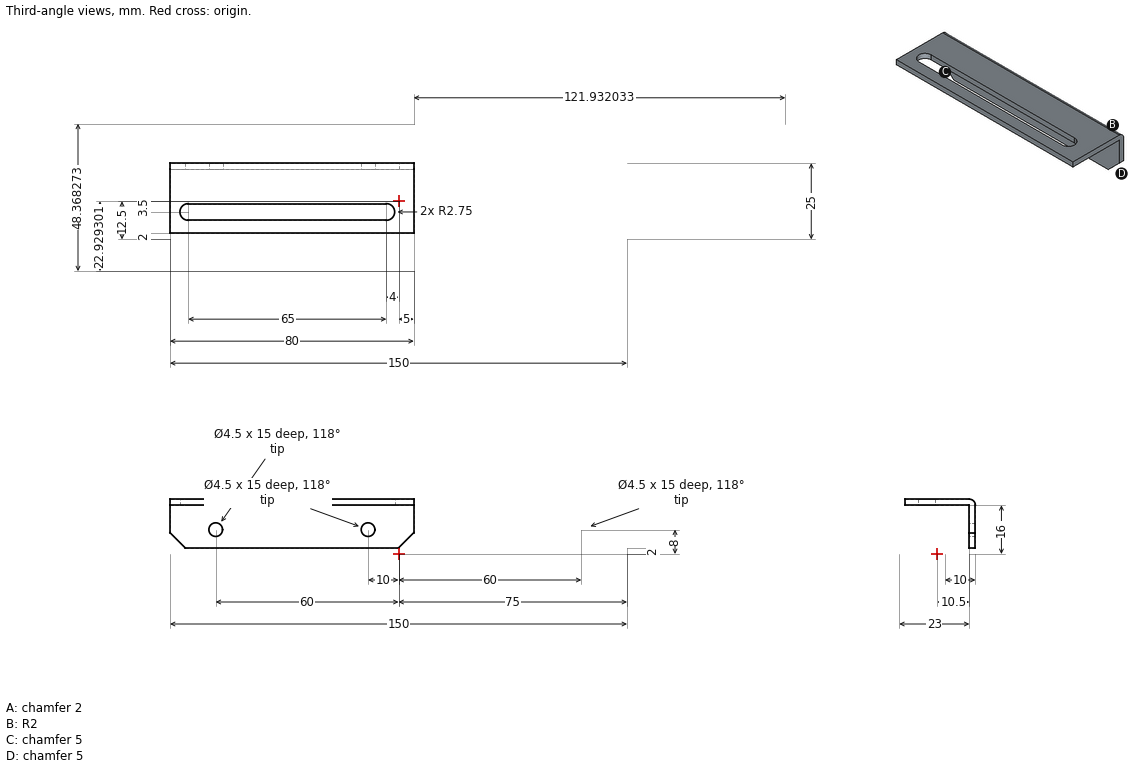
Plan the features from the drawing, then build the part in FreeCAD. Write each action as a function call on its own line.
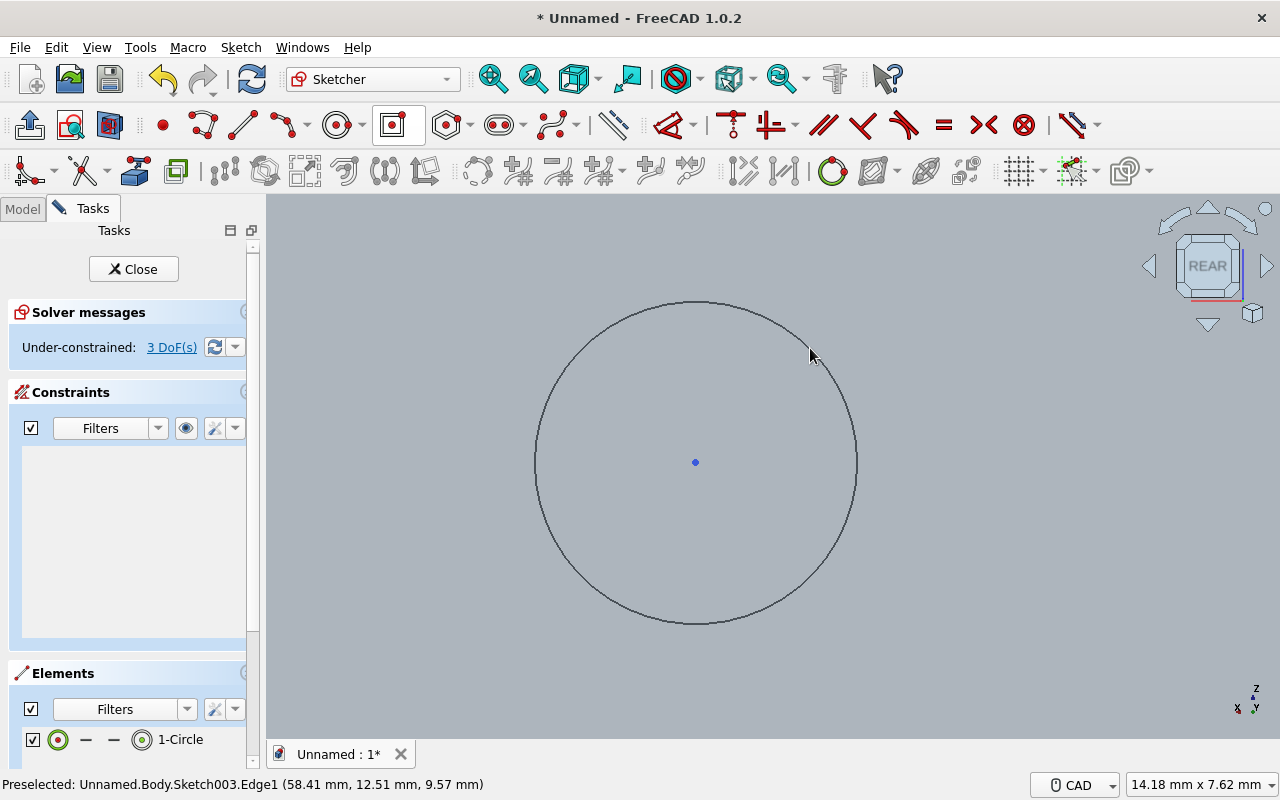
click(668, 126)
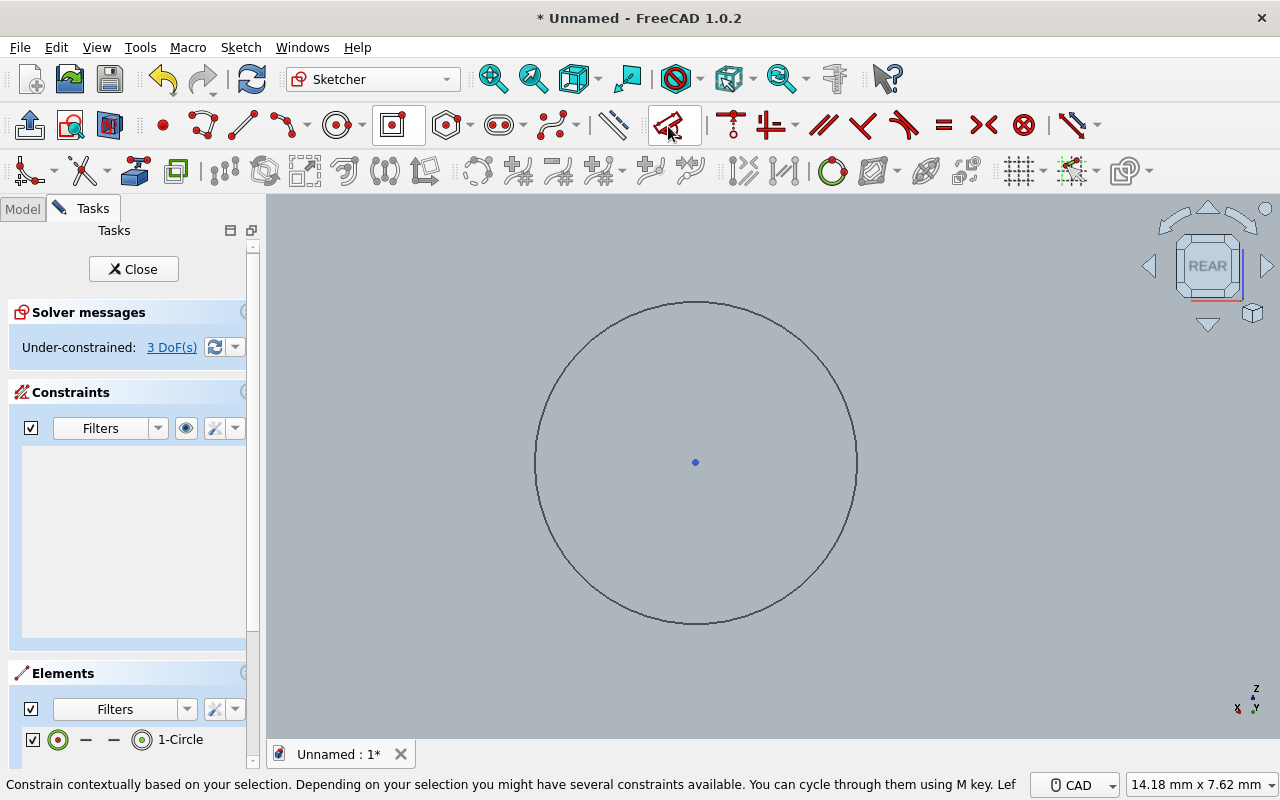
click(810, 349)
click(833, 326)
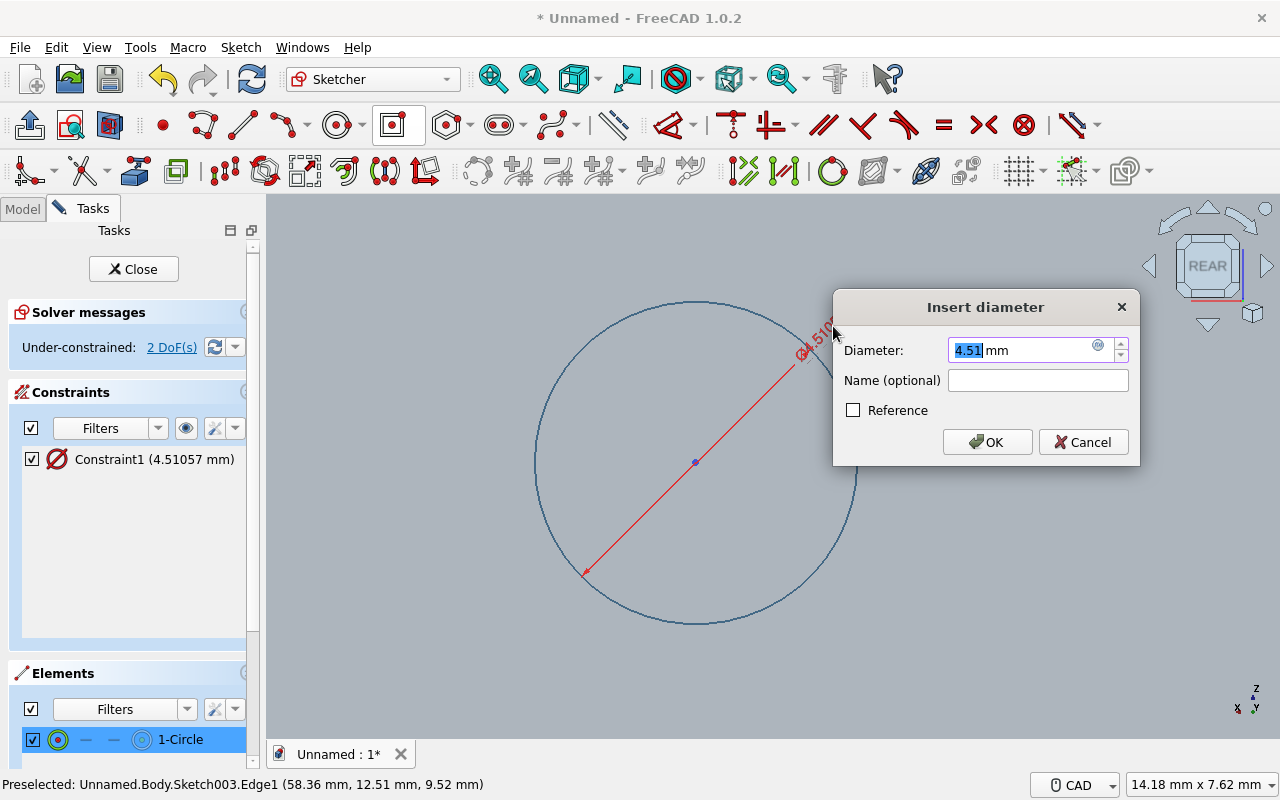
text(4.5)
key(Return)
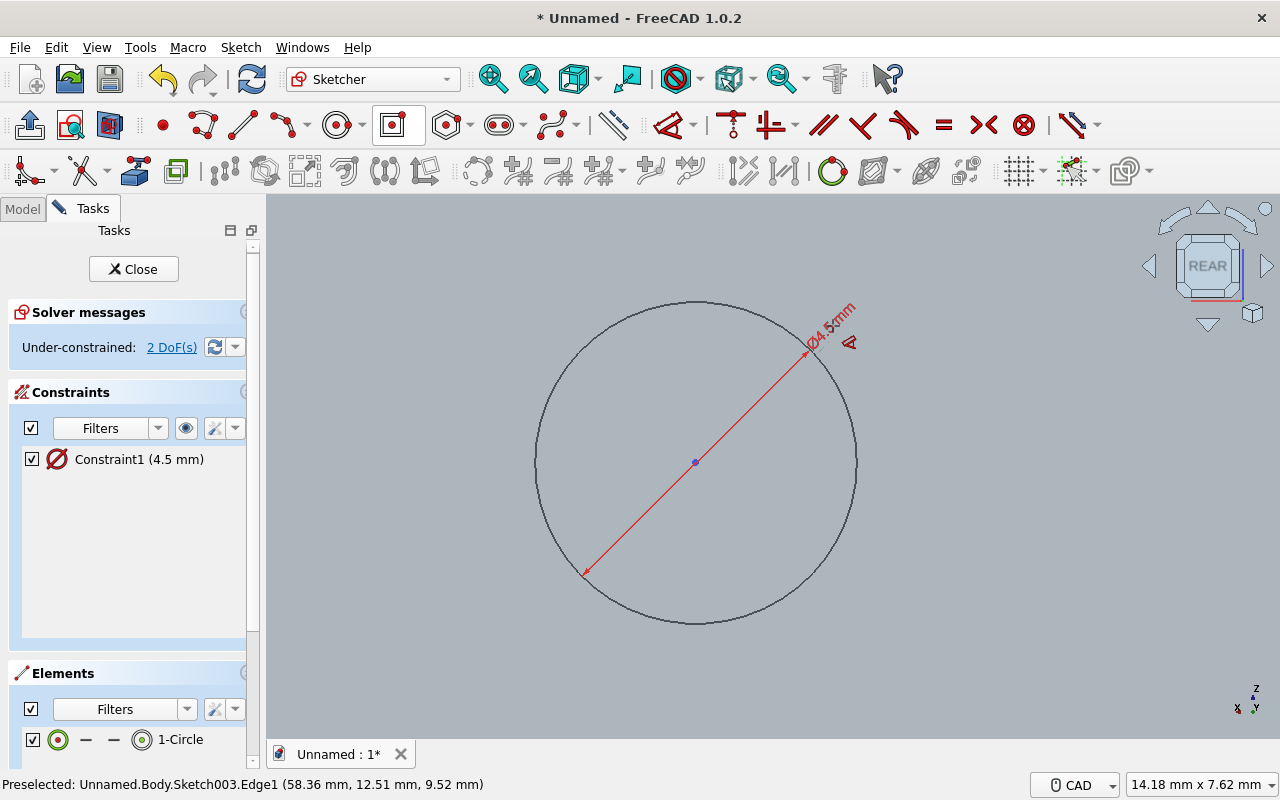
click(696, 463)
click(662, 587)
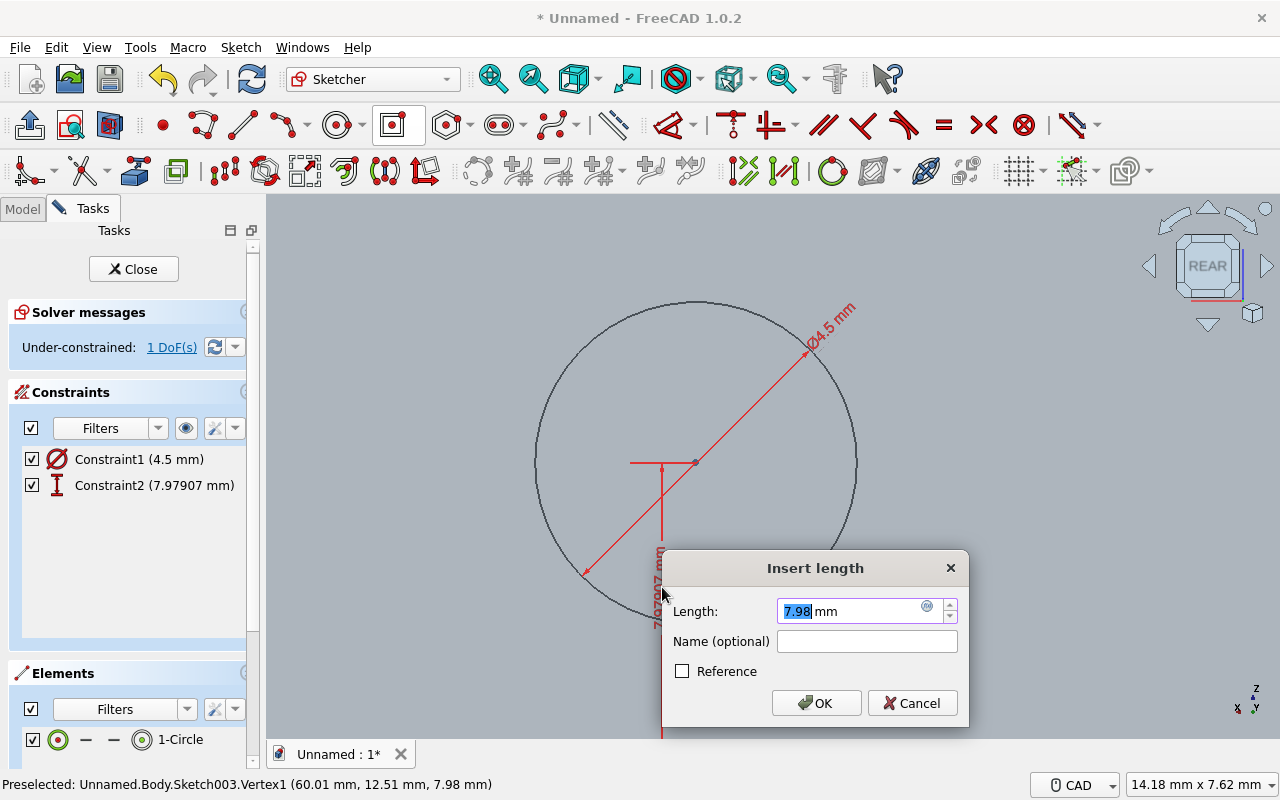
text(8)
key(Return)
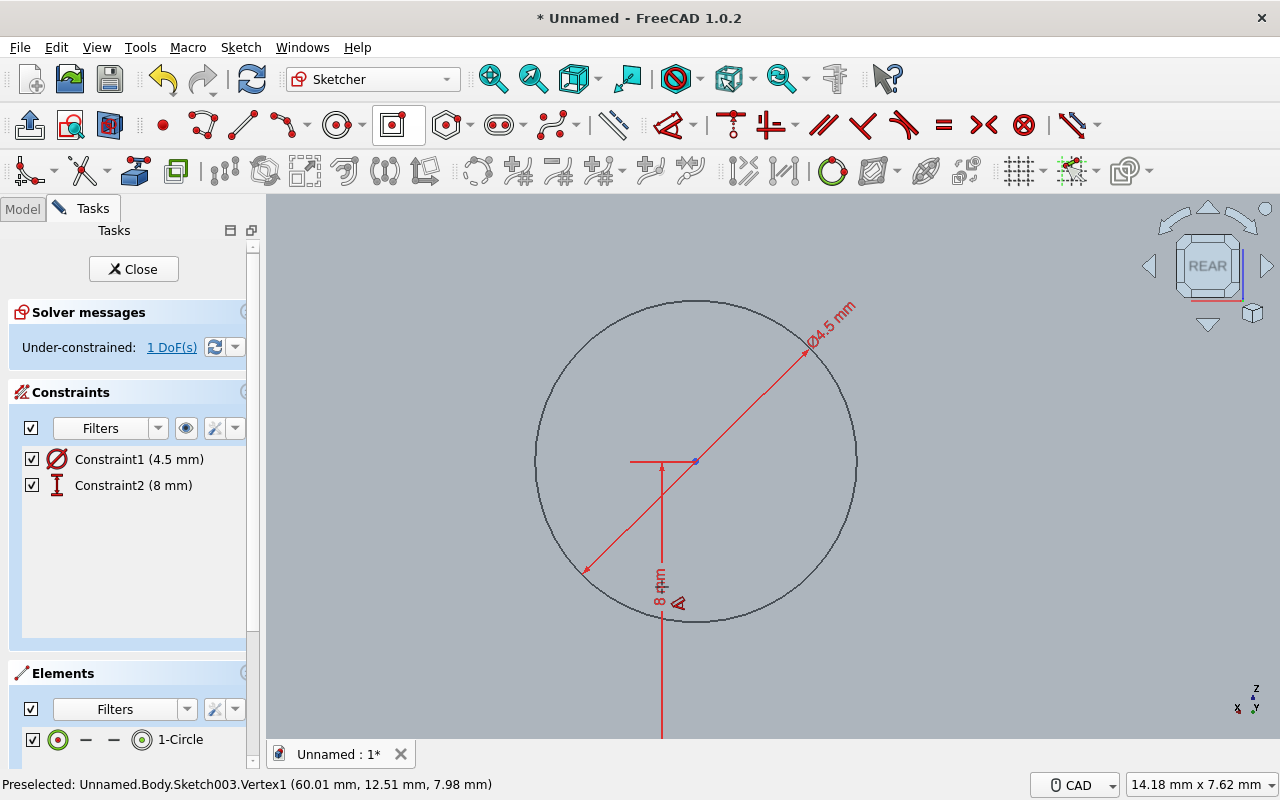
click(696, 462)
click(906, 428)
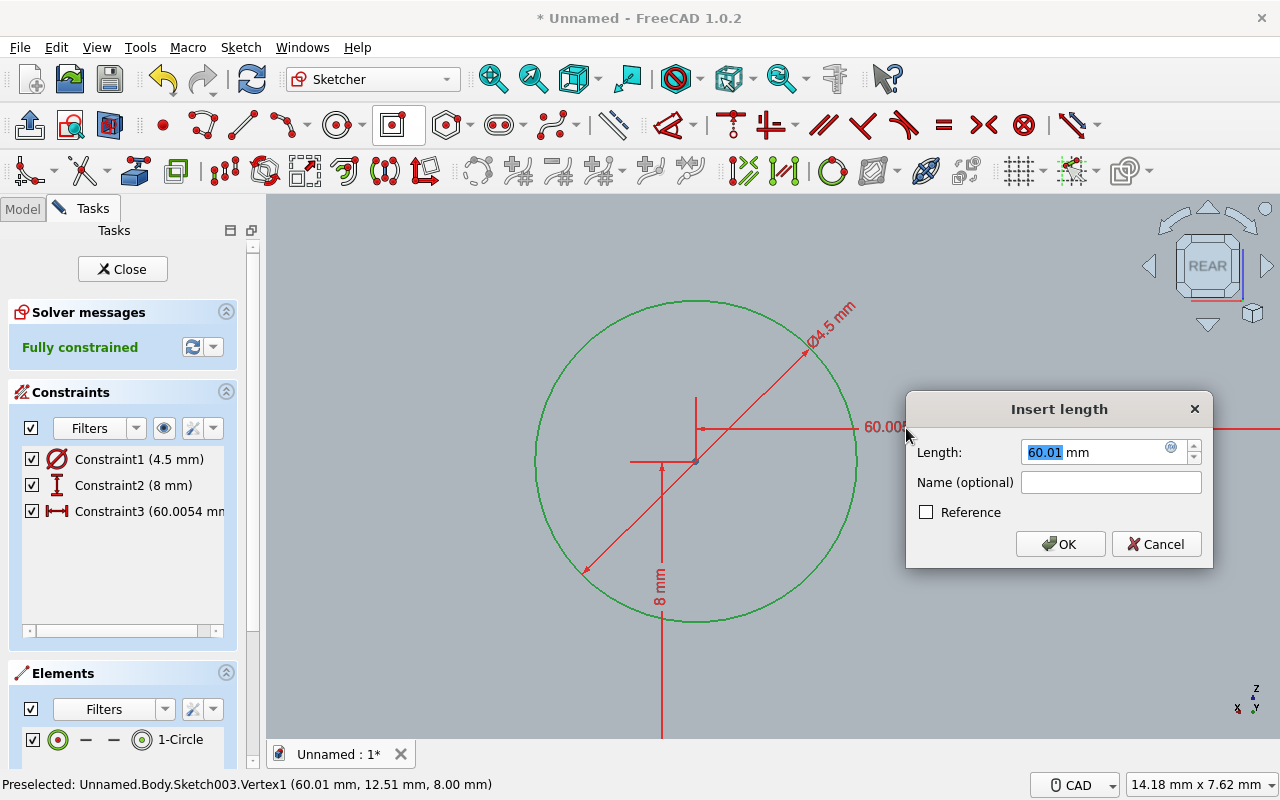
text(60)
key(Return)
key(Escape)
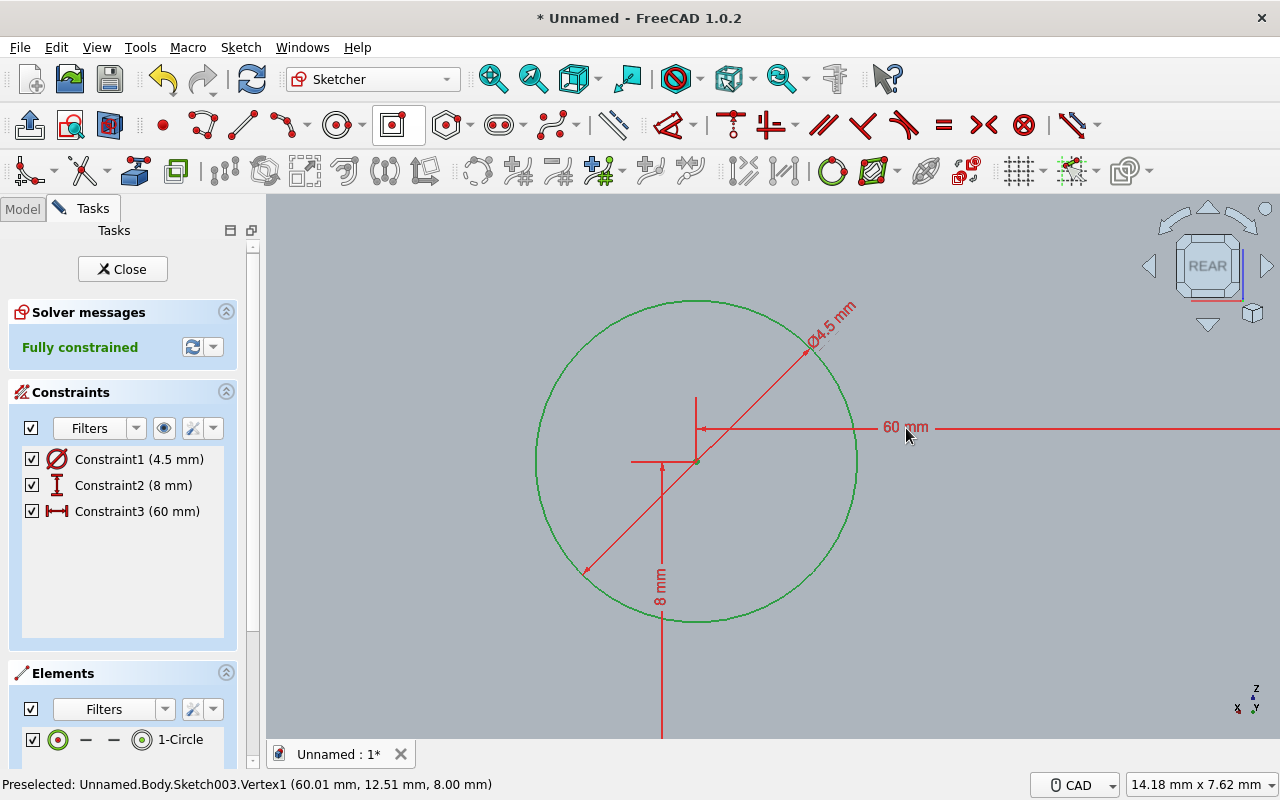
click(123, 269)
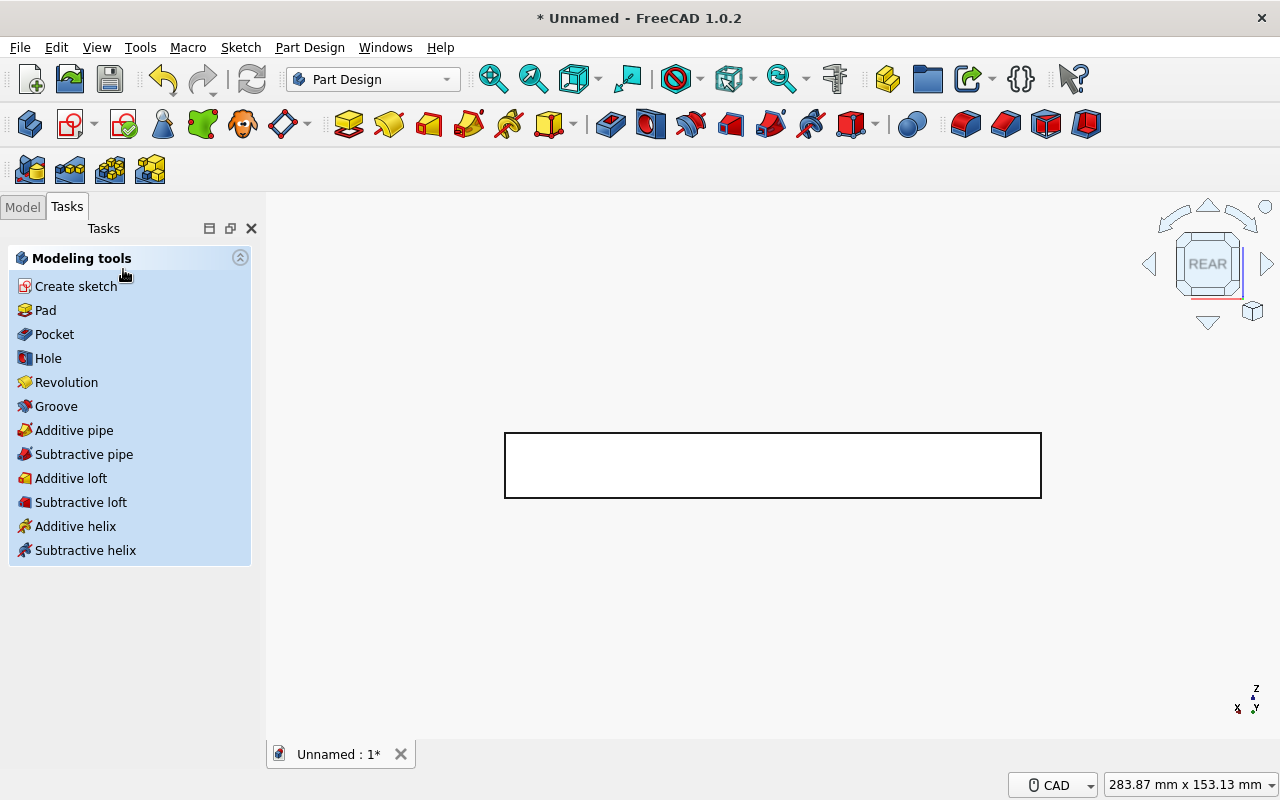
click(652, 124)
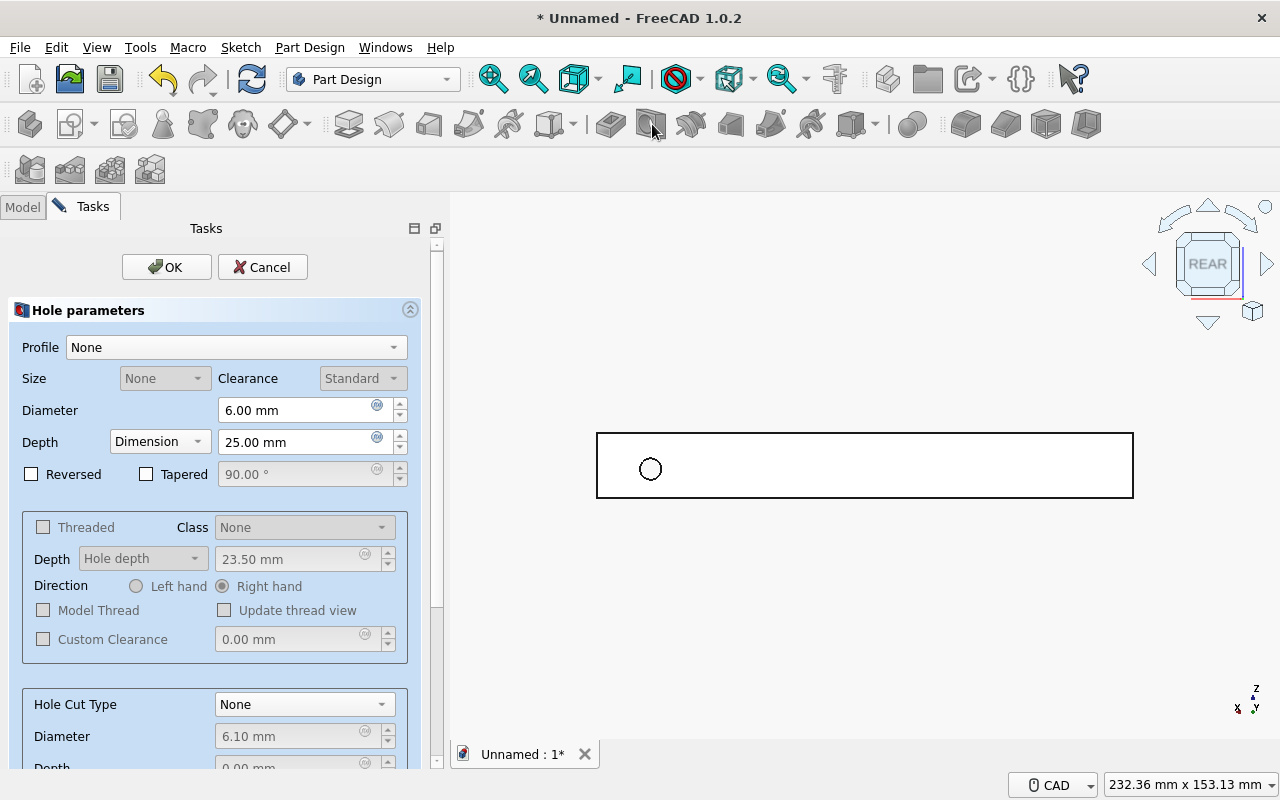
triple_click(305, 410)